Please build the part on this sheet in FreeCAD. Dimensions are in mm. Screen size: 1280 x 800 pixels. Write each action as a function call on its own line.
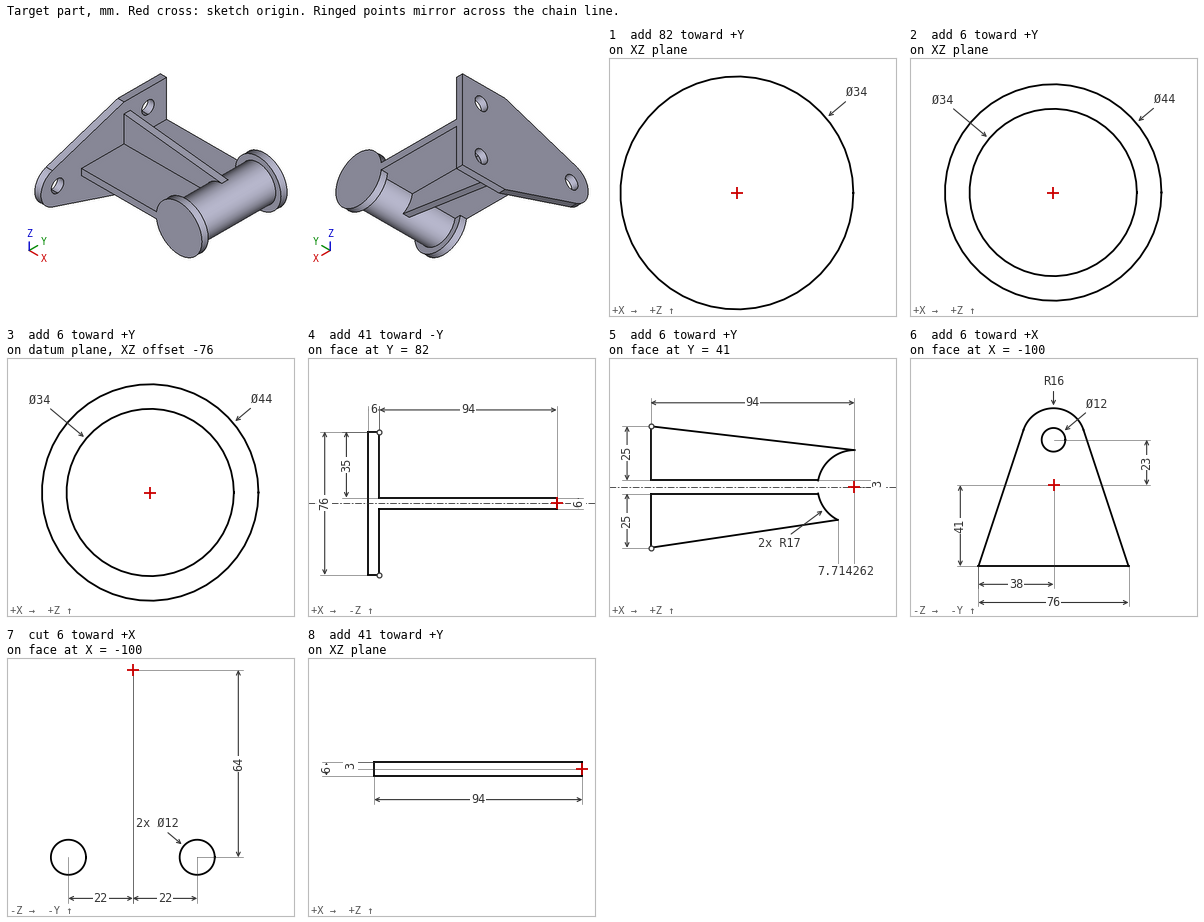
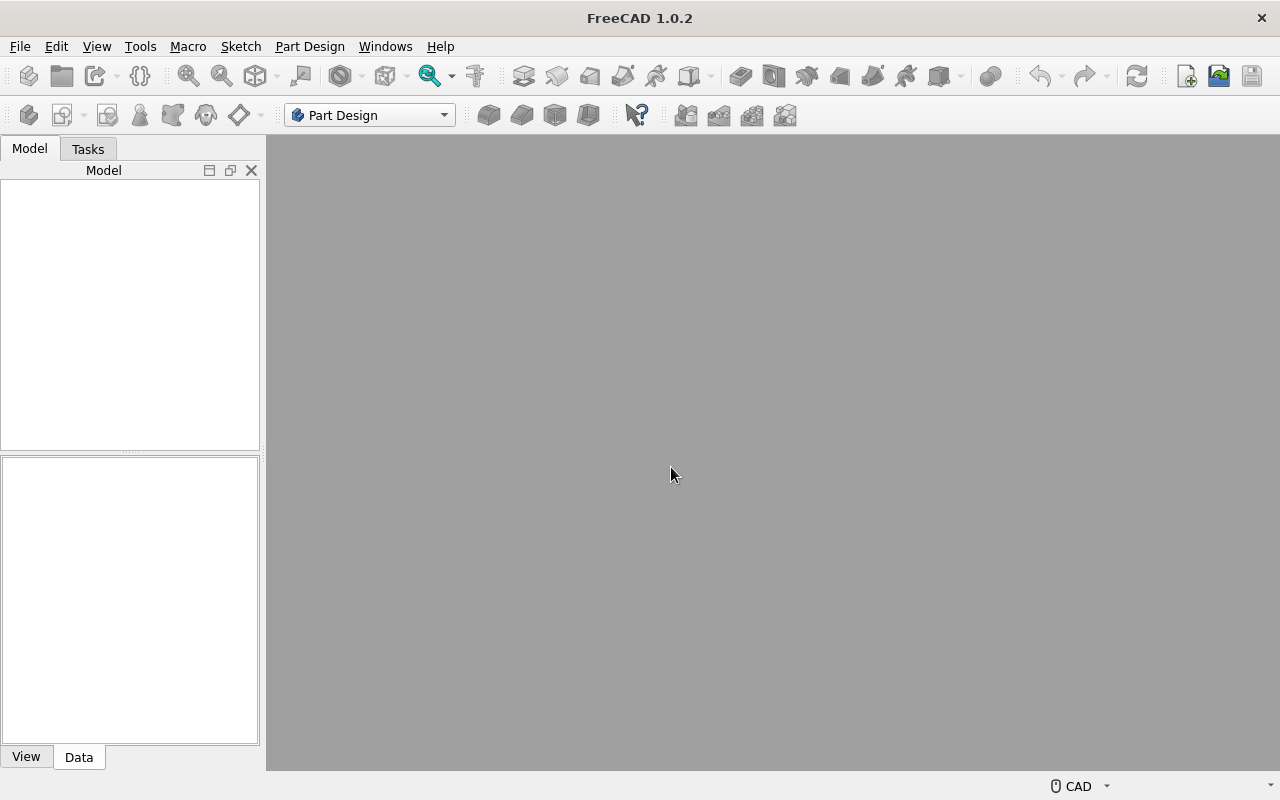
click(1186, 76)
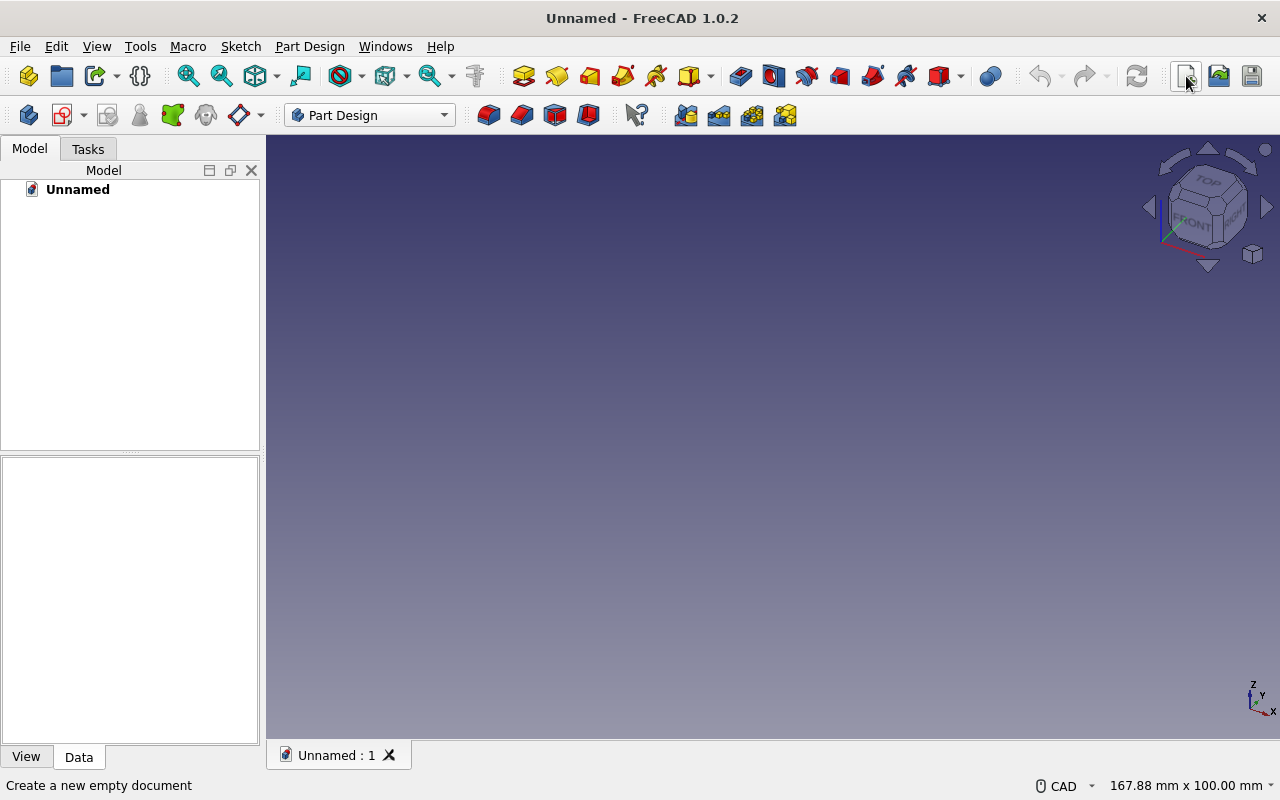
click(62, 116)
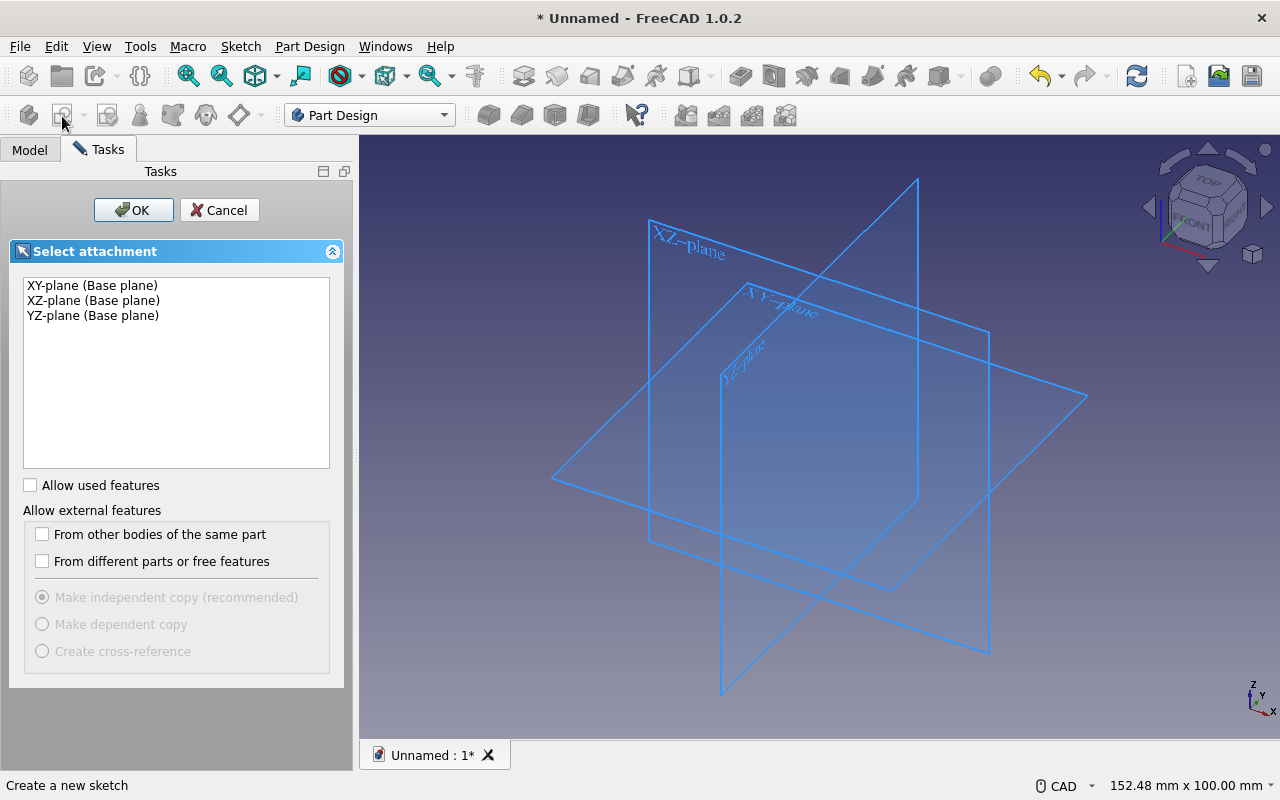
click(84, 300)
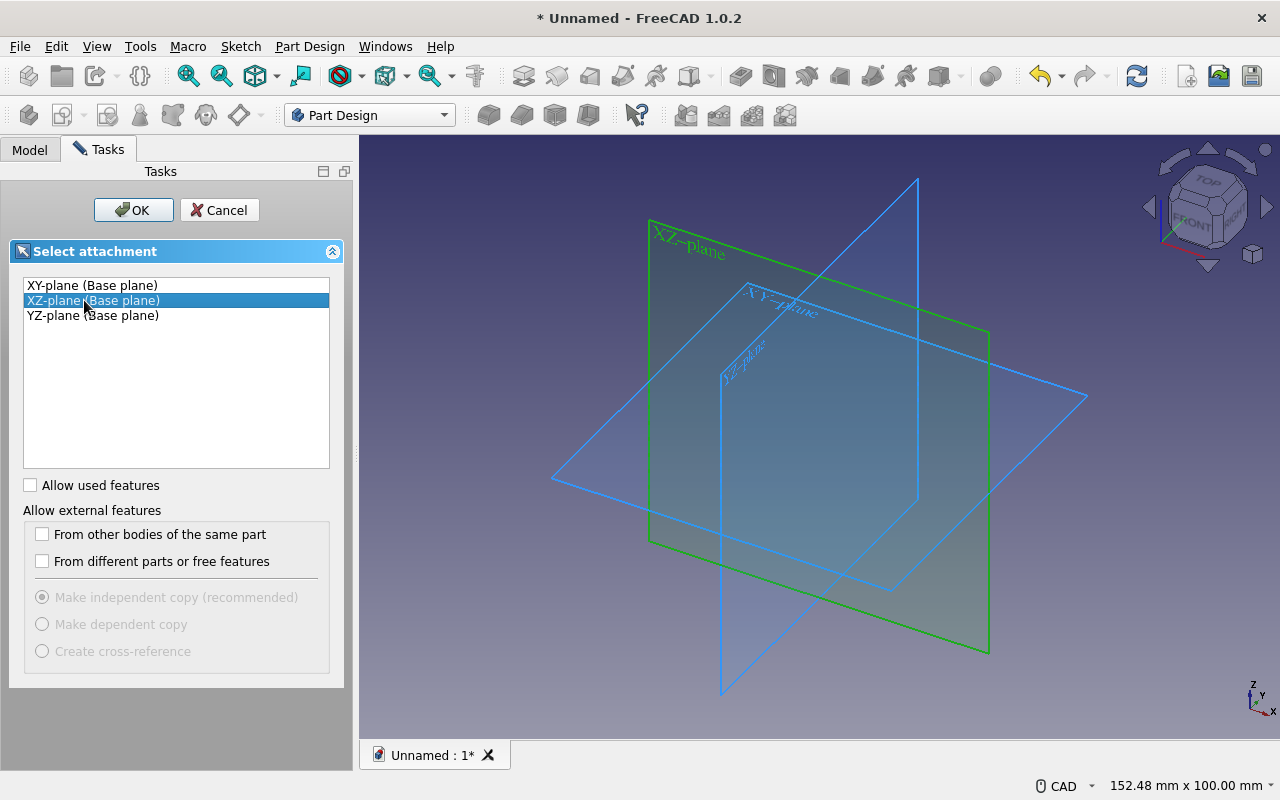
click(134, 210)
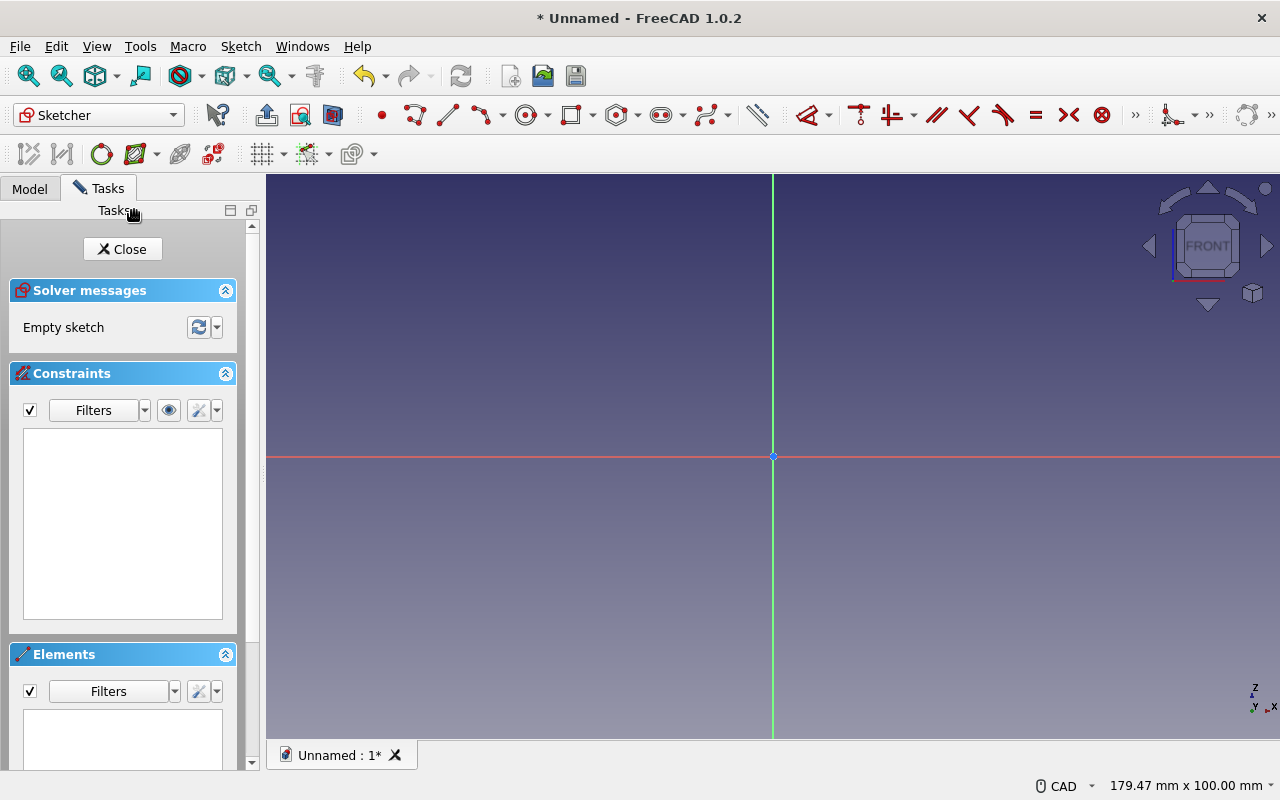
scroll(856, 456, up, 3)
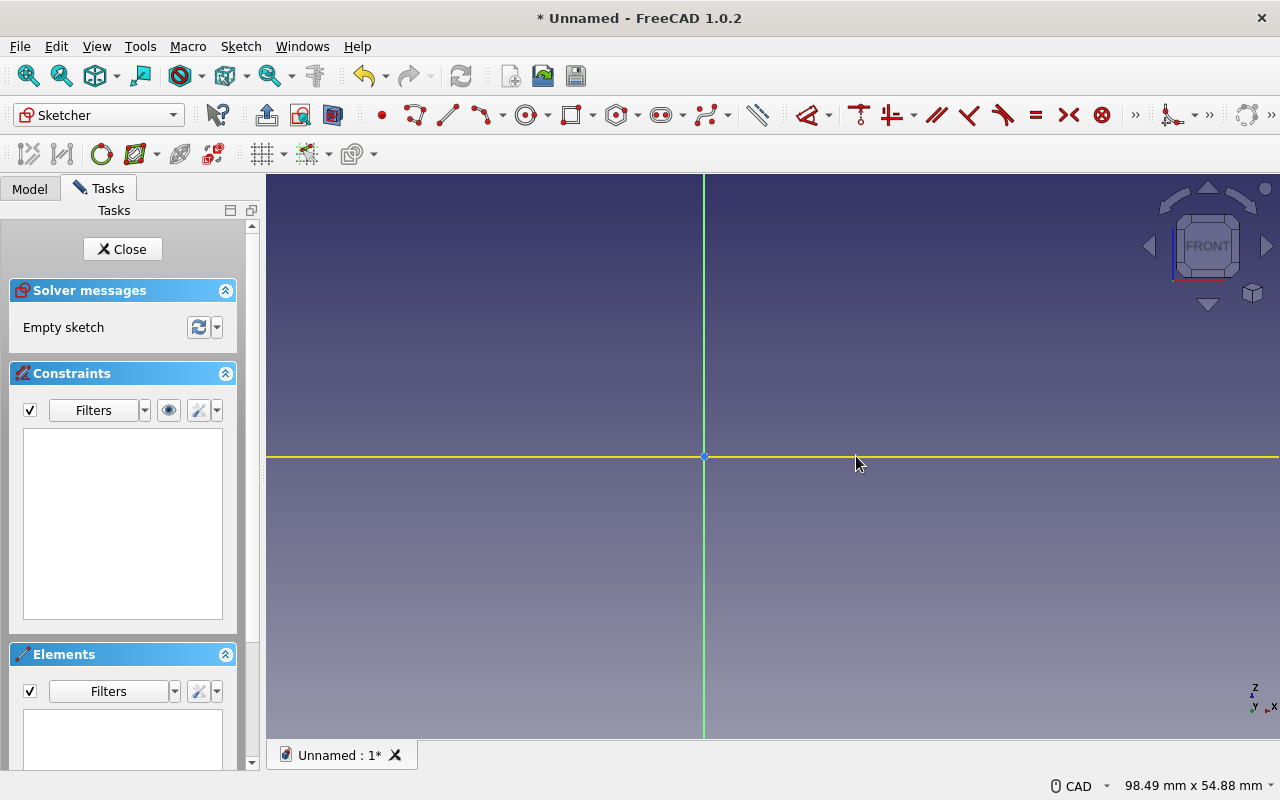
click(526, 116)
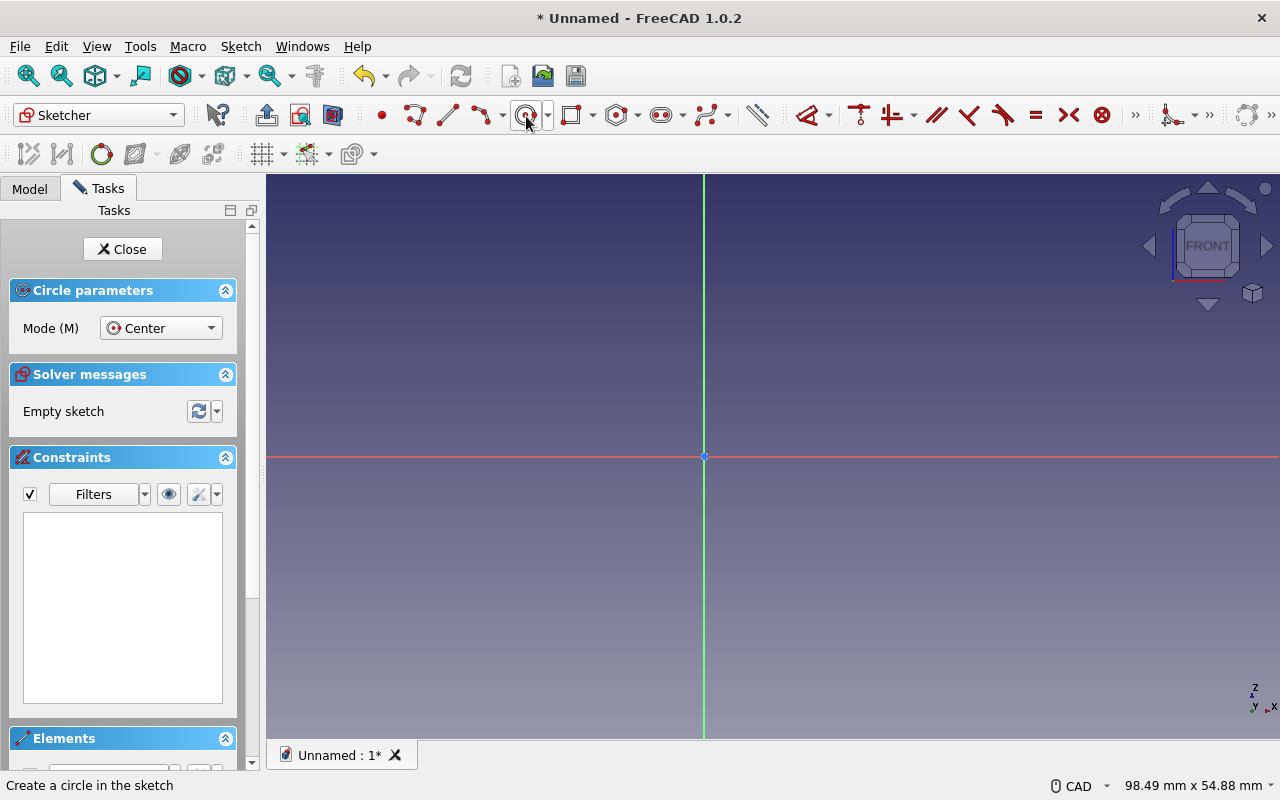
click(704, 456)
click(828, 333)
key(Escape)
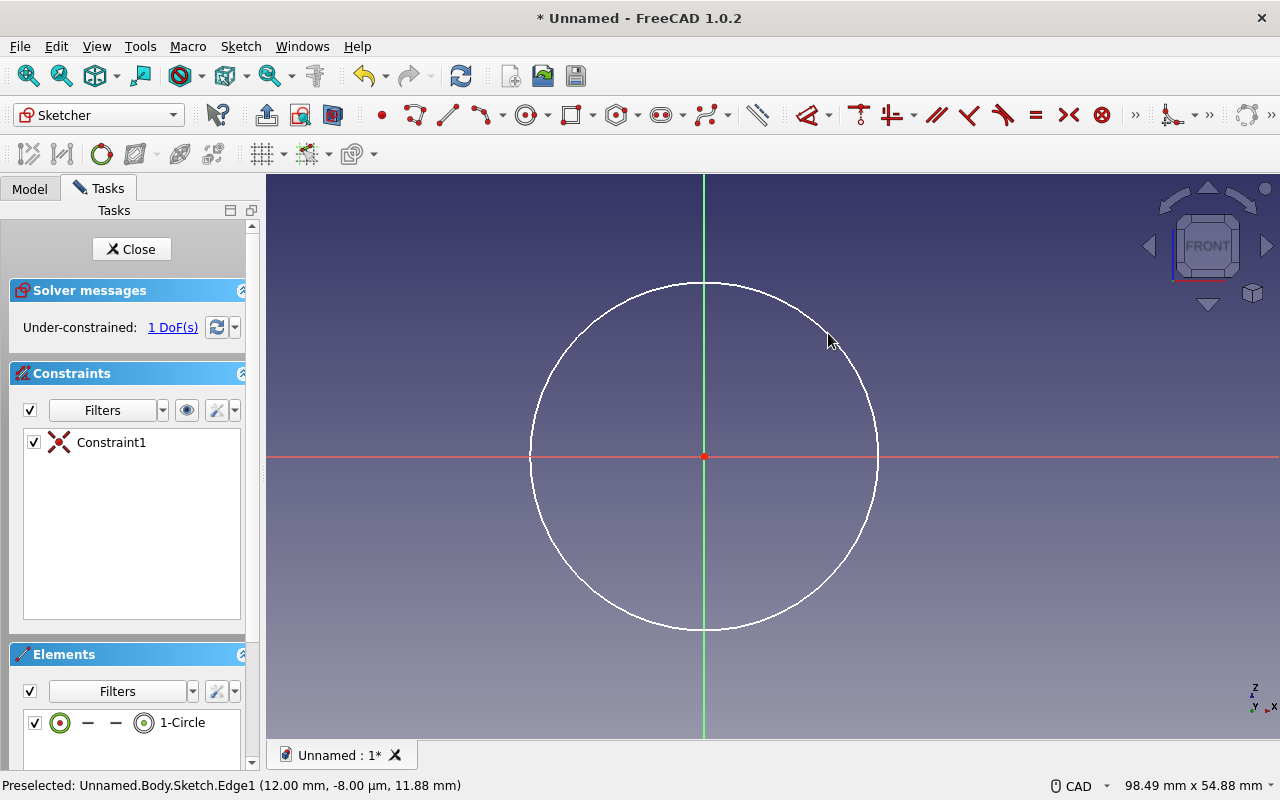
click(806, 116)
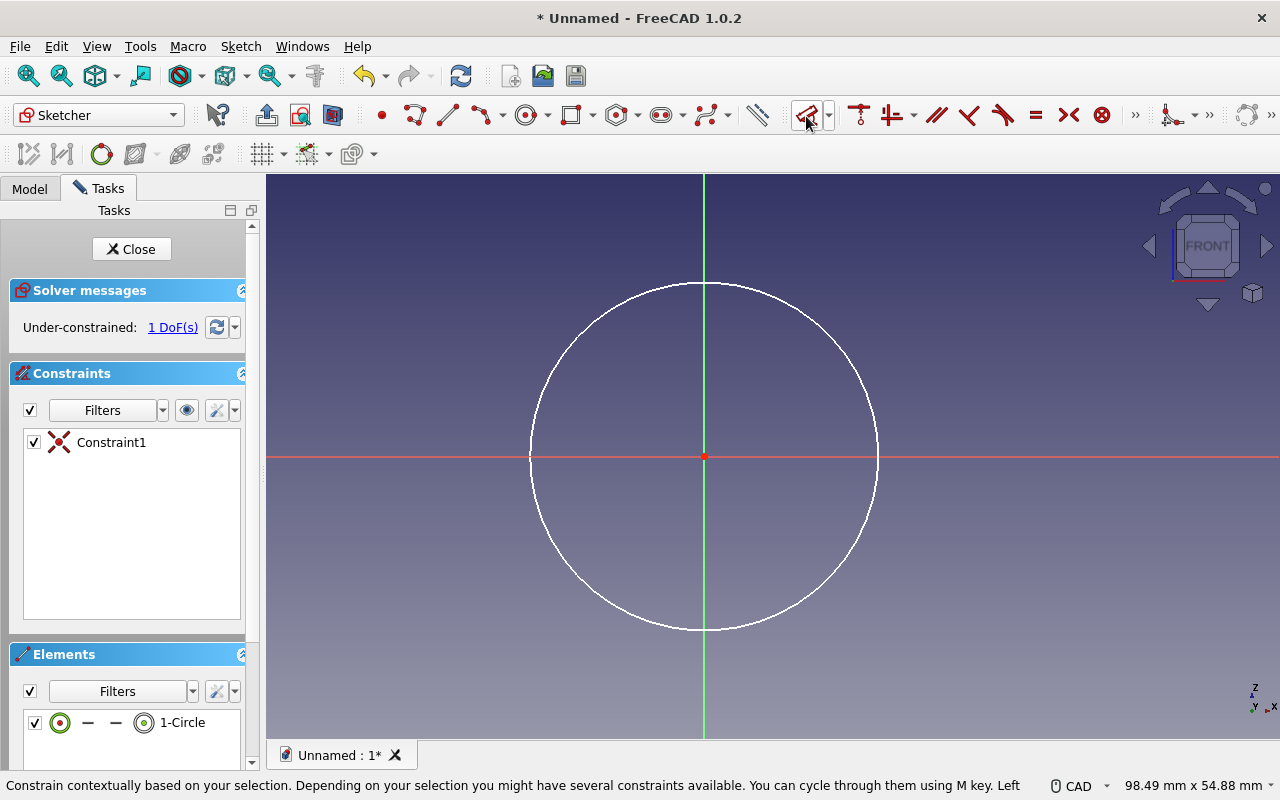
click(827, 333)
click(850, 310)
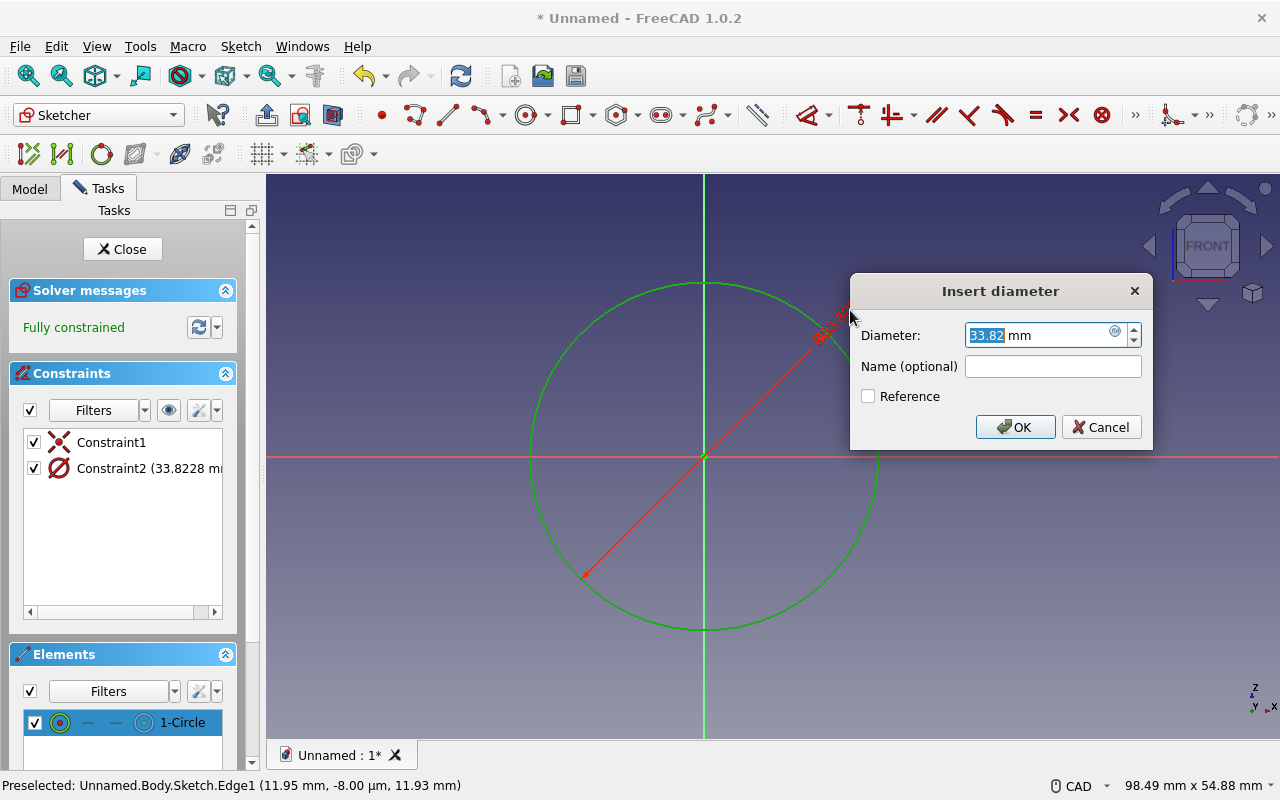
text(34)
key(Return)
key(Escape)